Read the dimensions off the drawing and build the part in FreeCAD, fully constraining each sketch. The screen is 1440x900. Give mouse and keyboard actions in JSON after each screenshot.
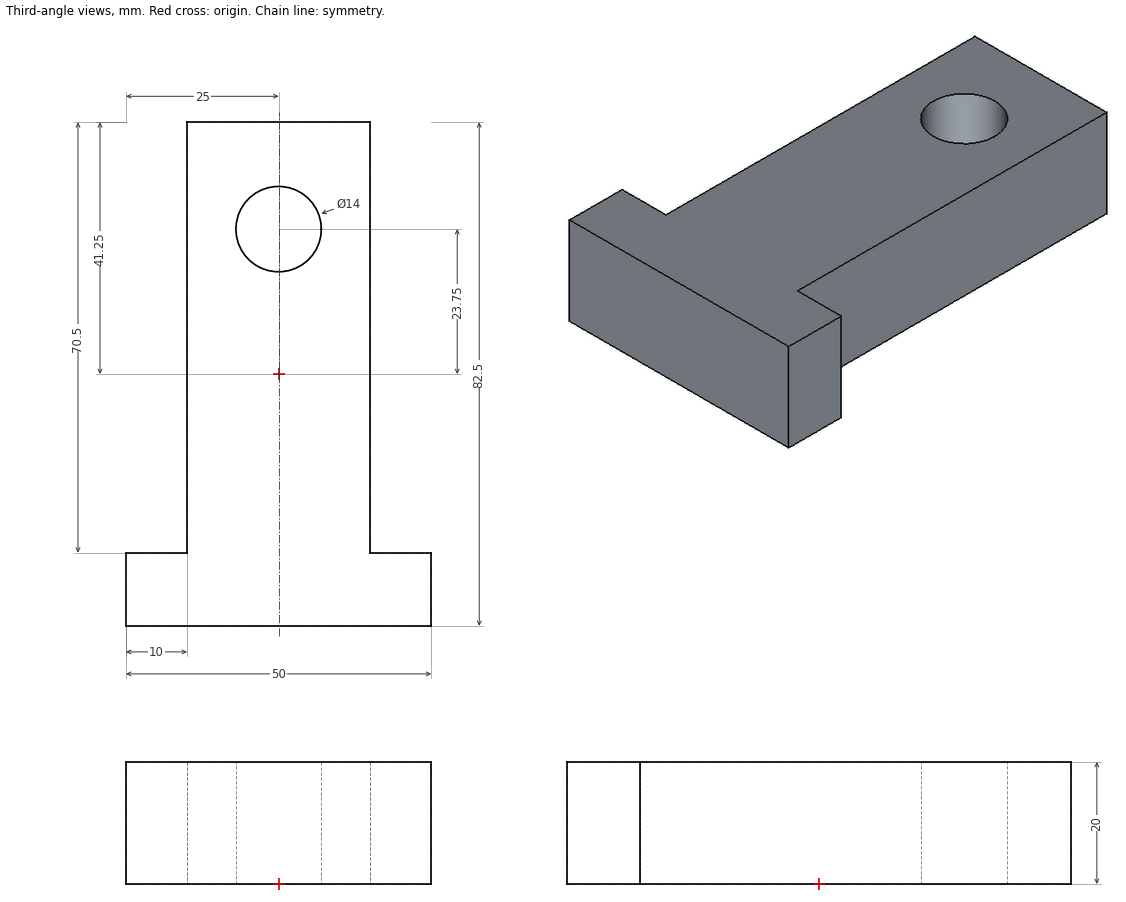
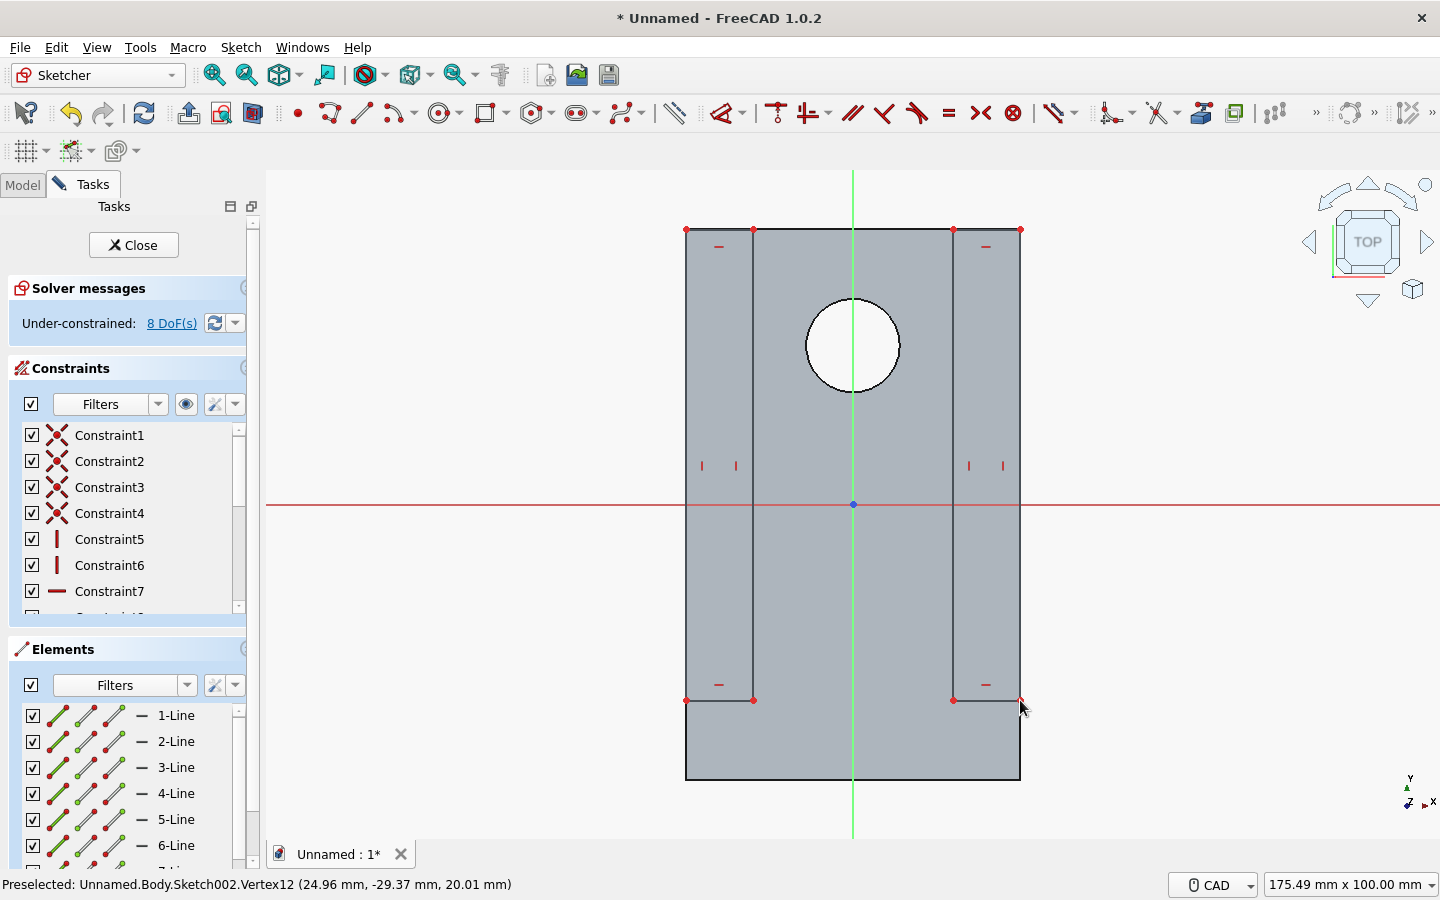
{"action": "left_click", "coordinate": [753, 230]}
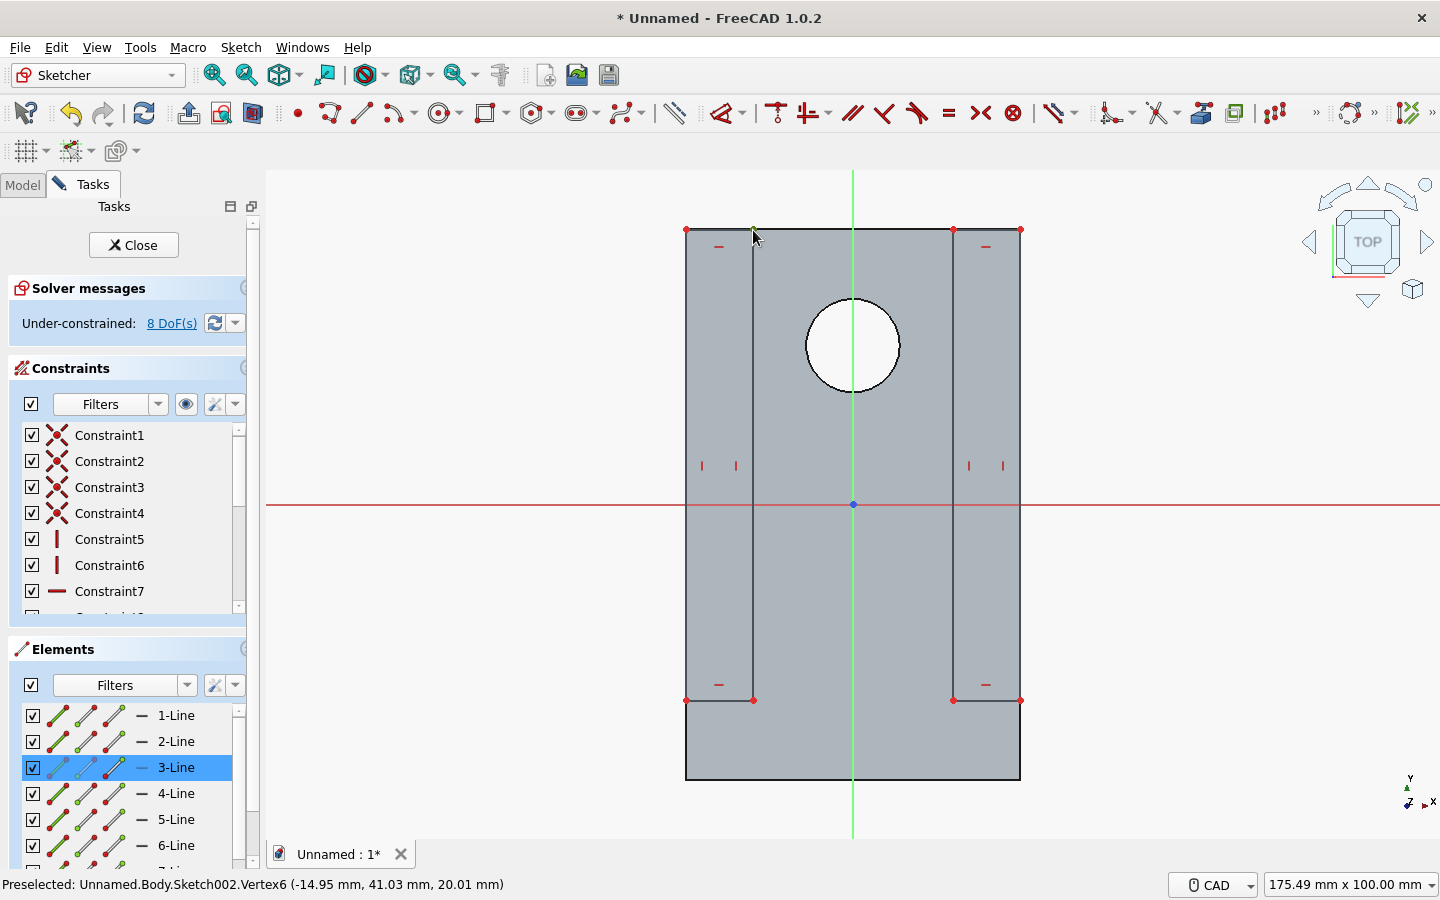
{"action": "left_click", "coordinate": [953, 230]}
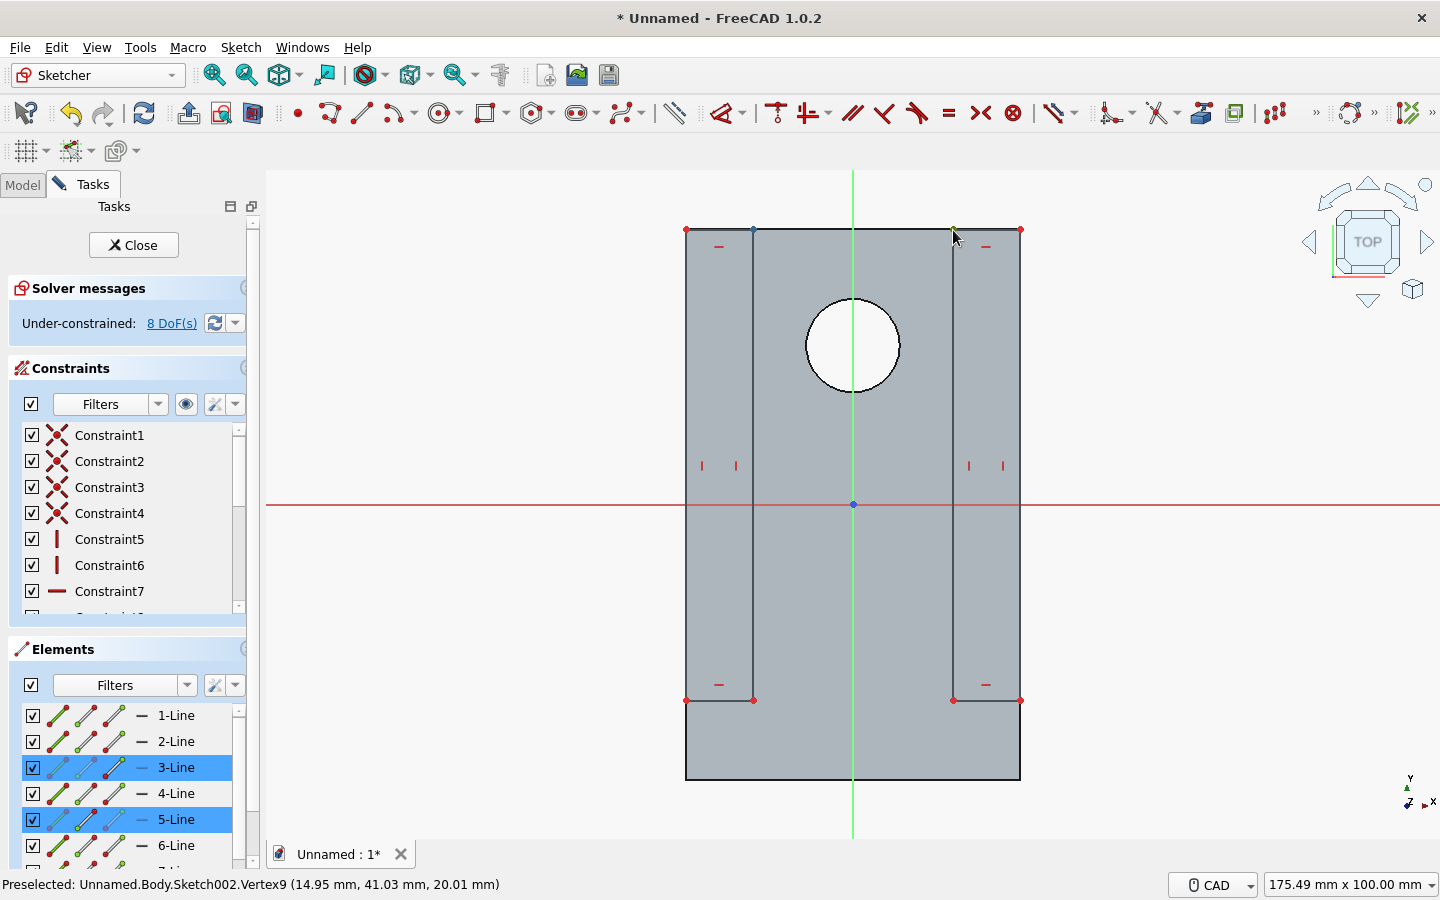
{"action": "left_click", "coordinate": [853, 767]}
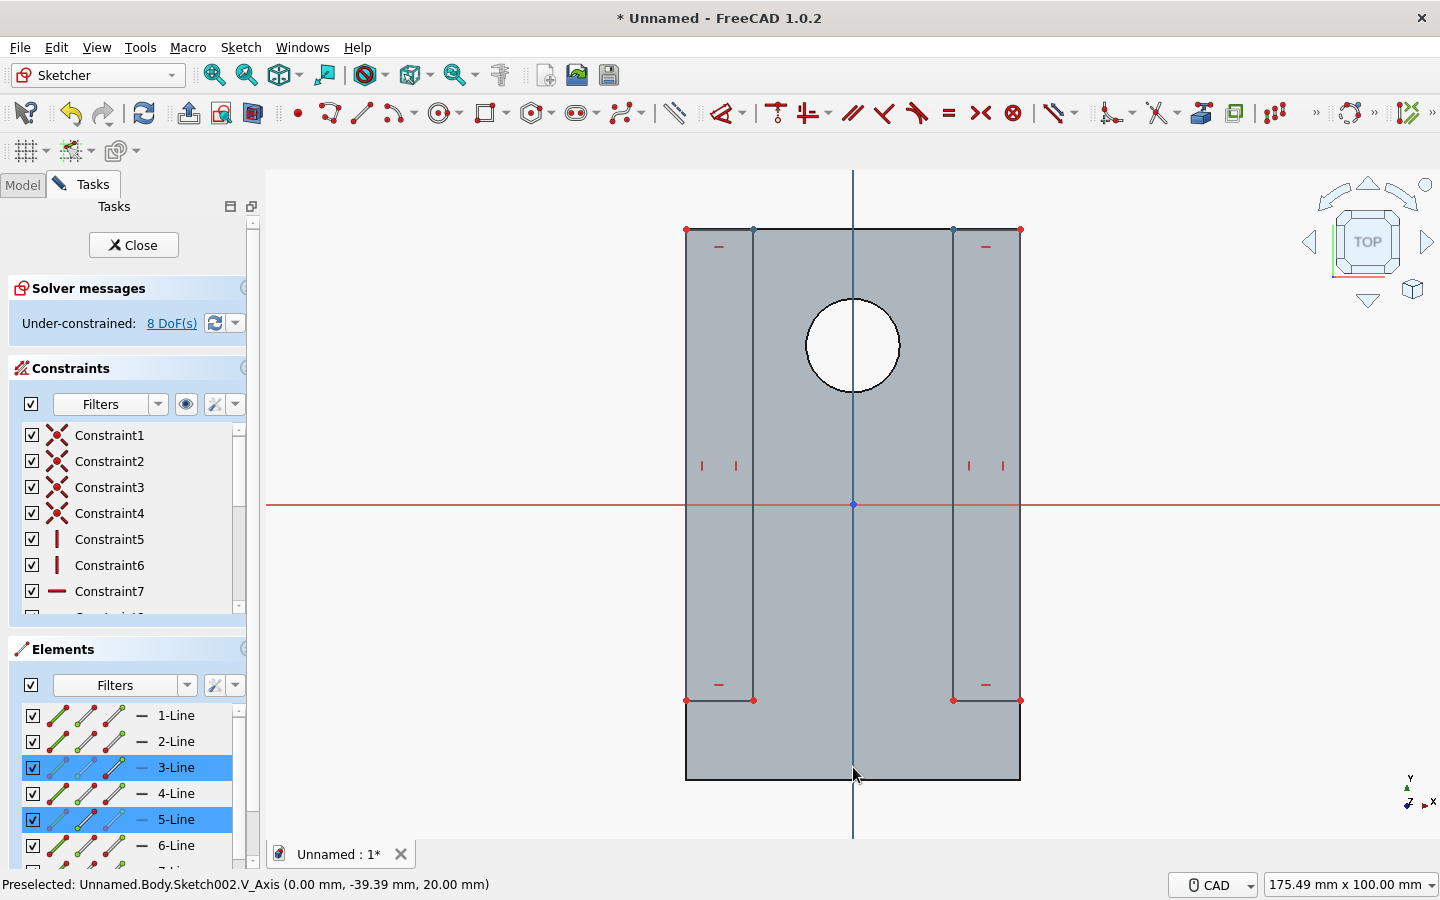
{"action": "left_click", "coordinate": [982, 114]}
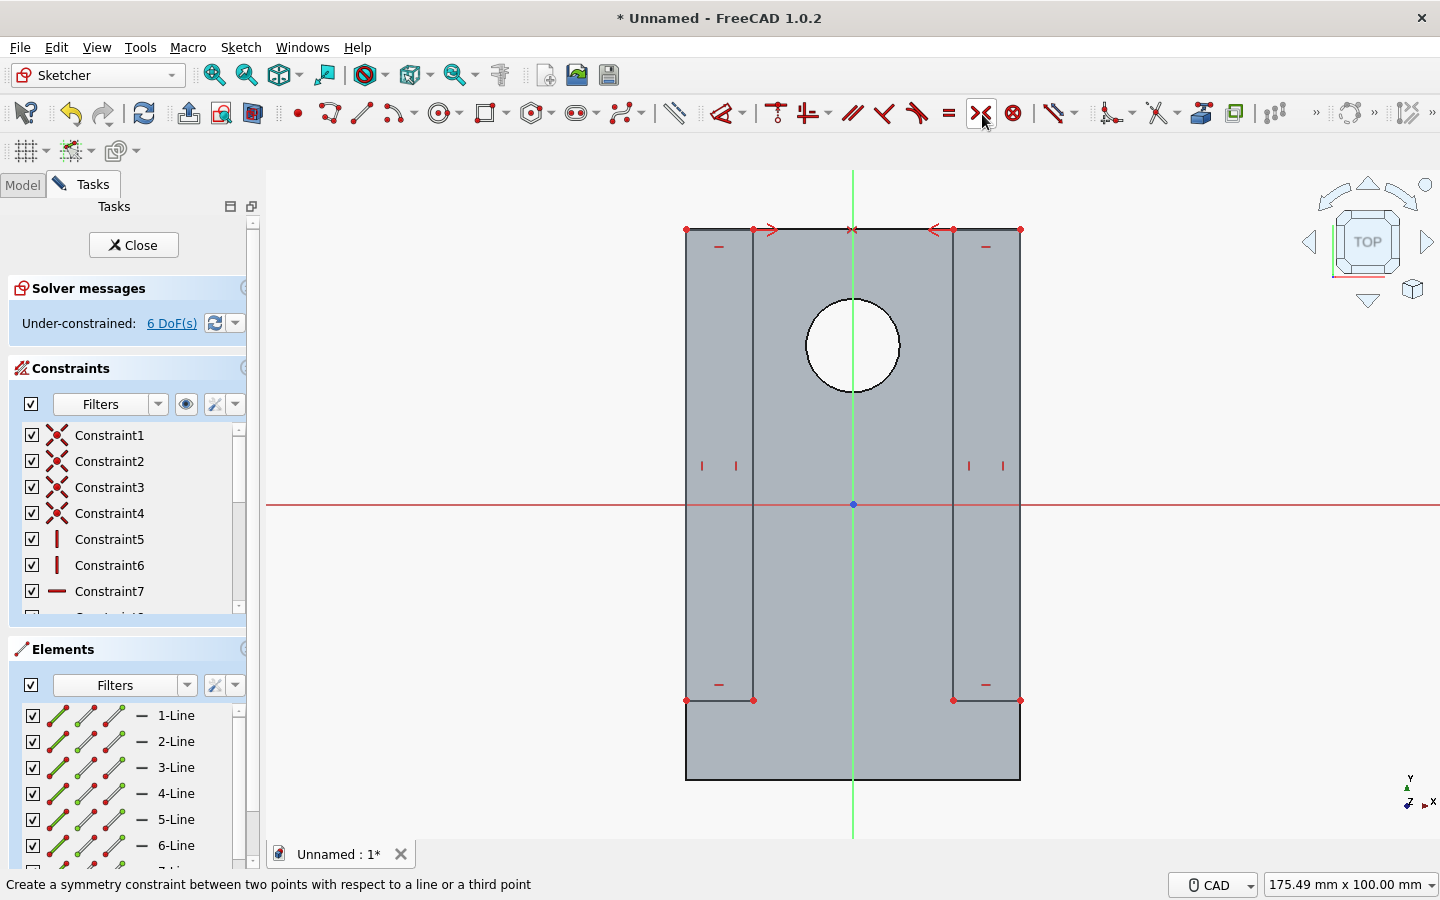
{"action": "left_click", "coordinate": [686, 701]}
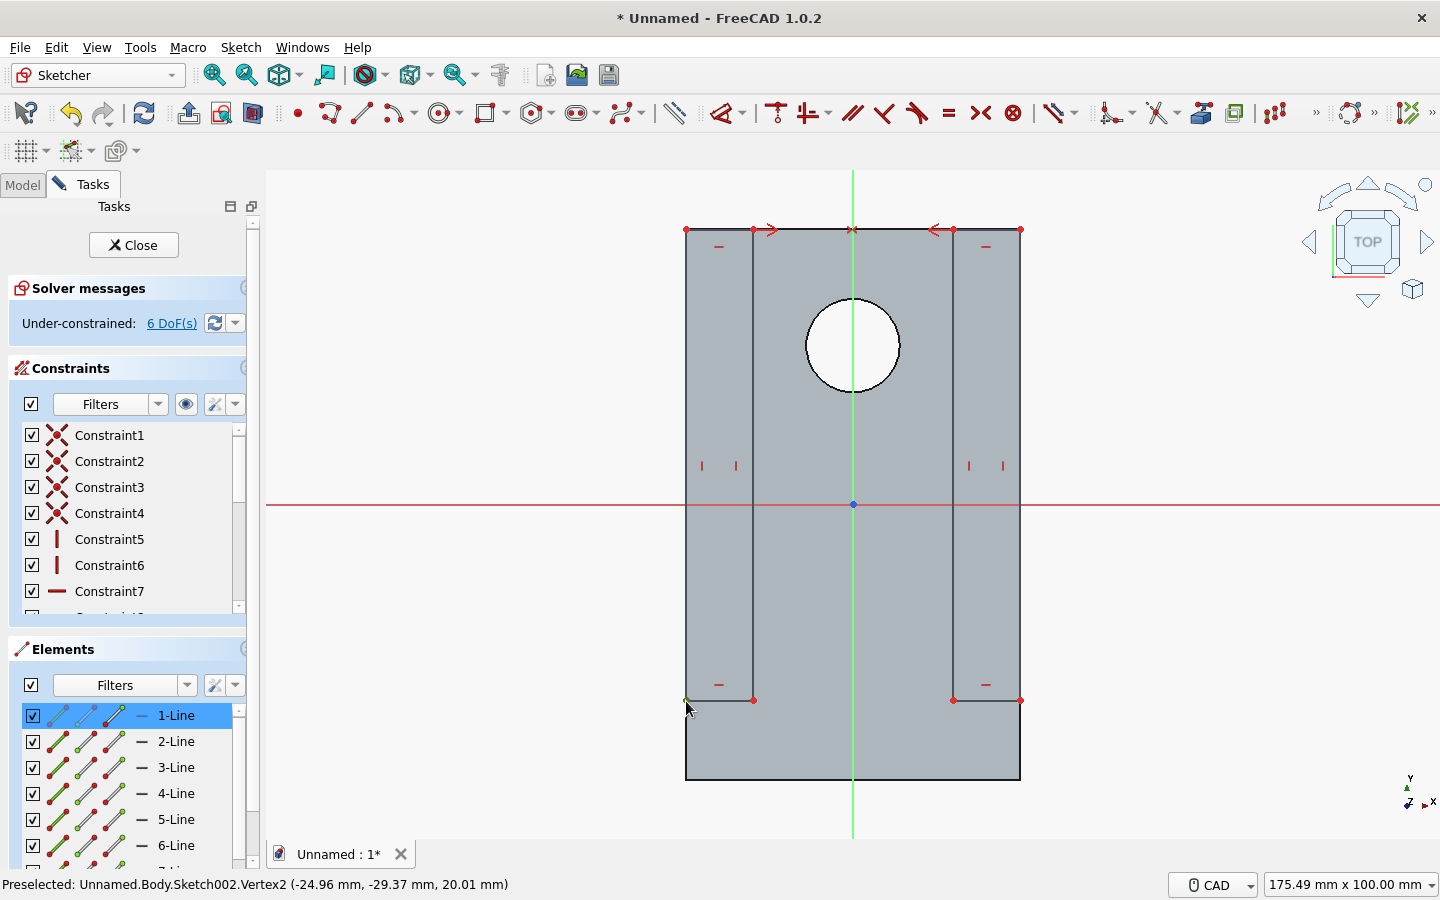
{"action": "left_click", "coordinate": [1020, 701]}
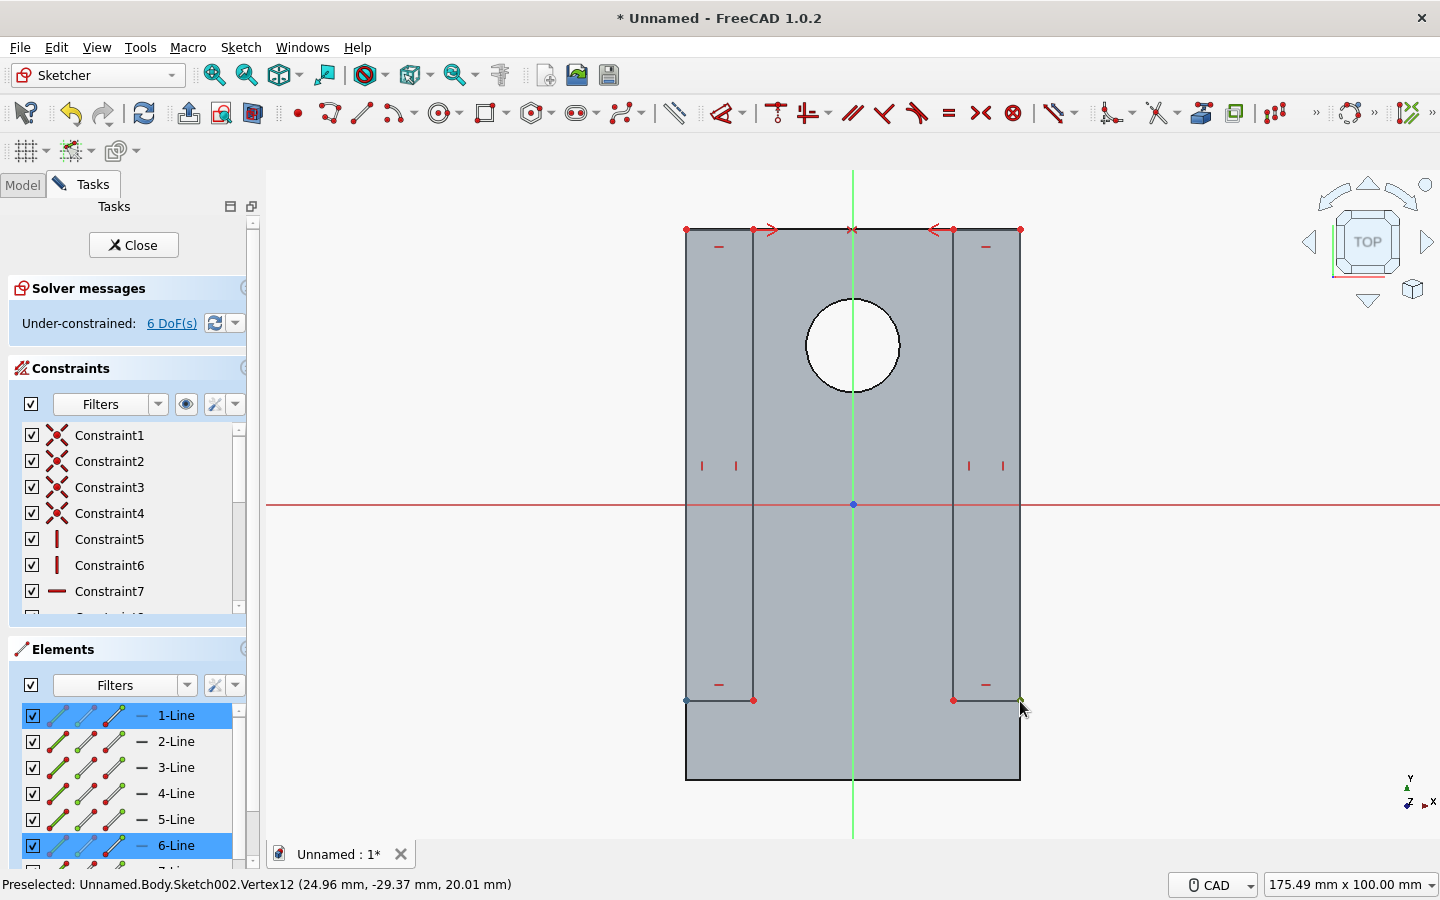
{"action": "left_click", "coordinate": [853, 767]}